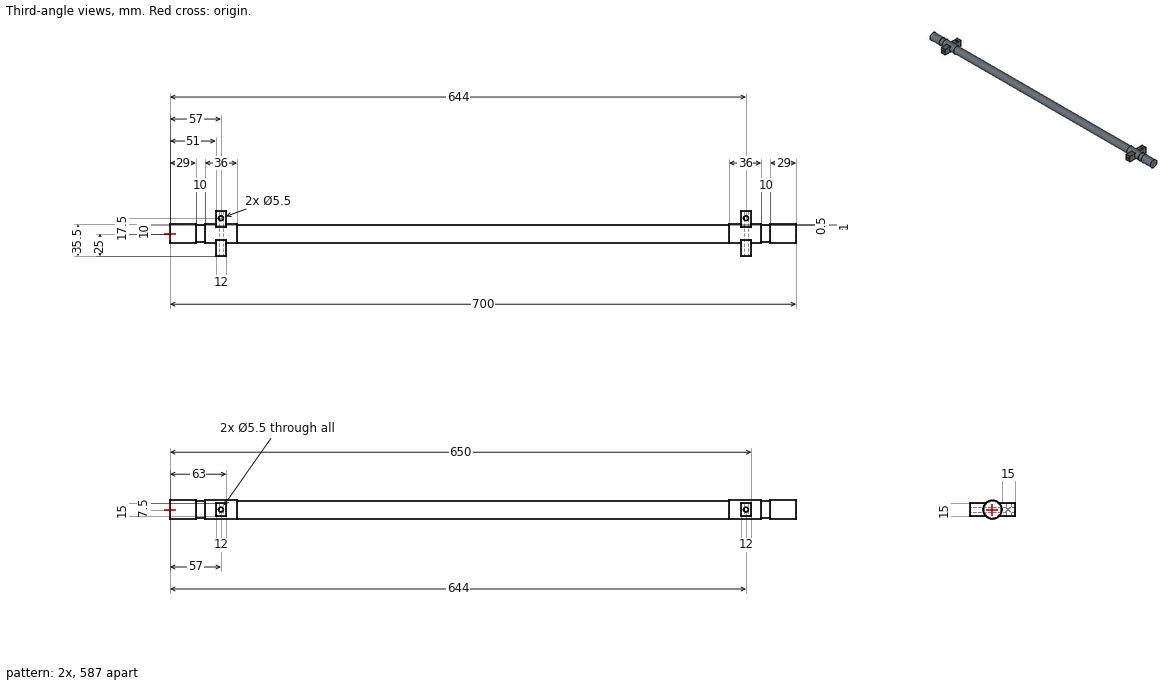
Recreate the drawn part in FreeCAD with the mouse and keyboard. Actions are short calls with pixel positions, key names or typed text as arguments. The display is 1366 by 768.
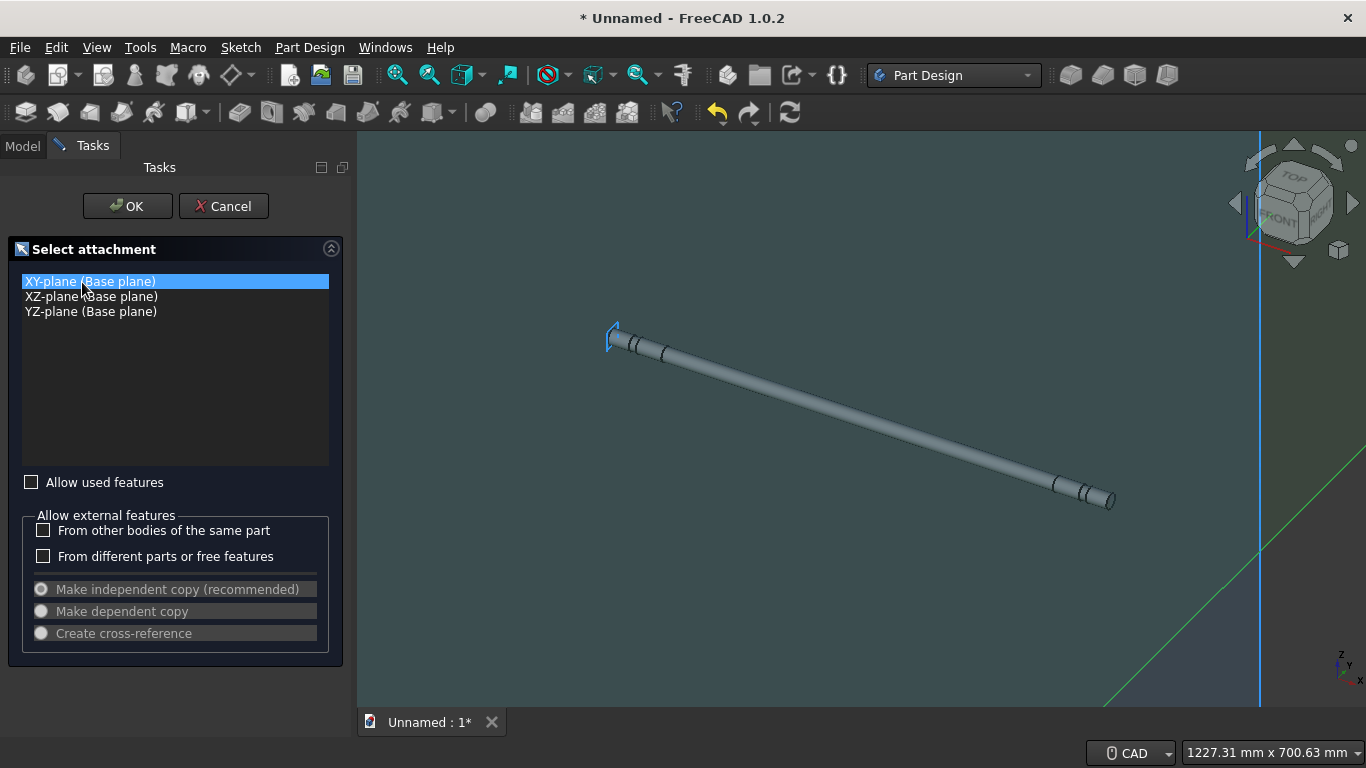
click(128, 206)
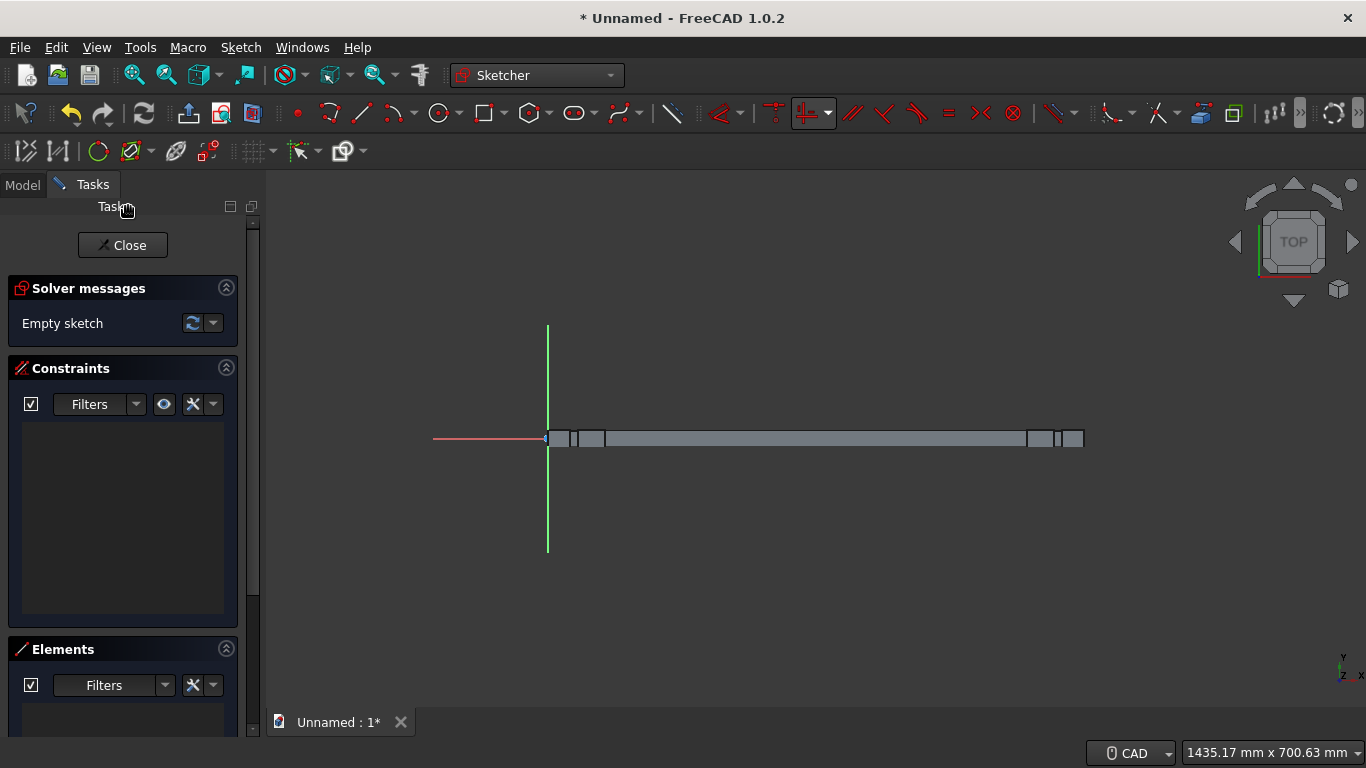
click(254, 114)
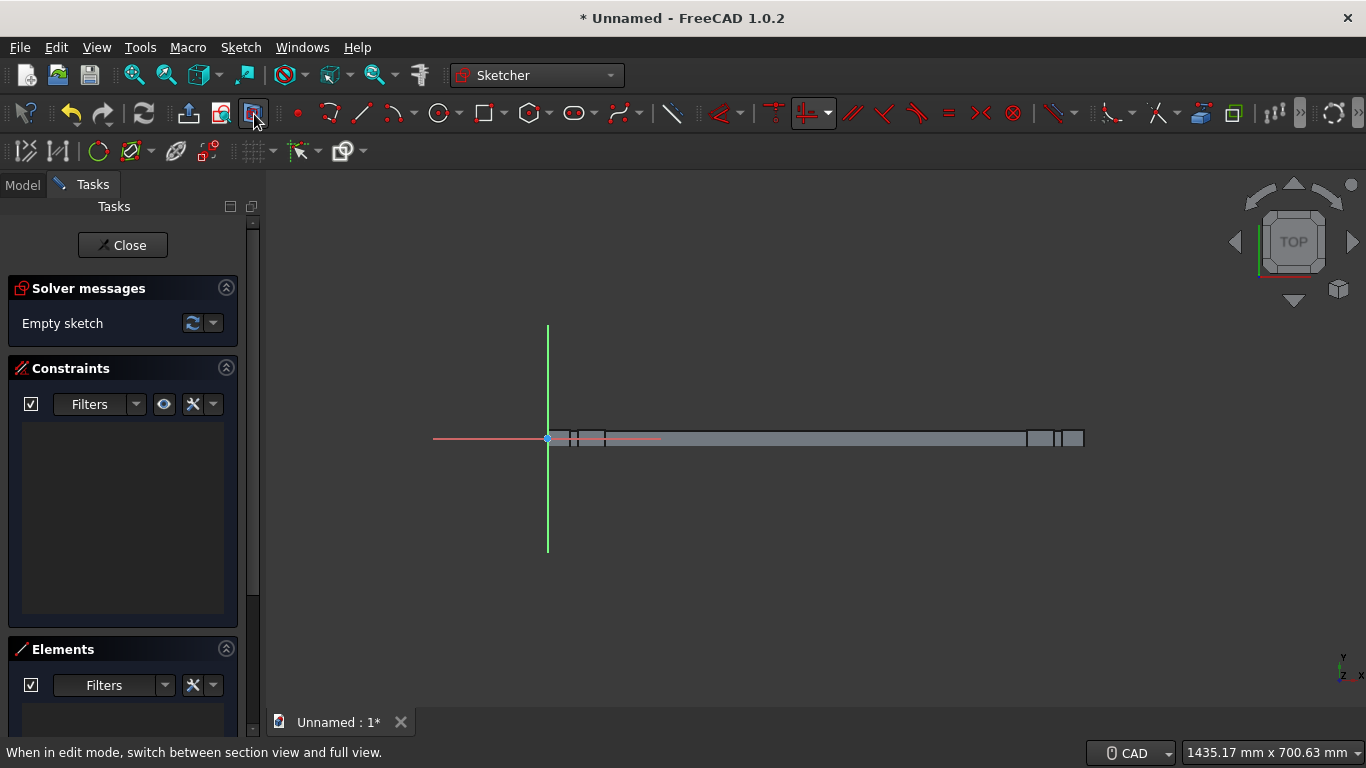
scroll(558, 445, up, 13)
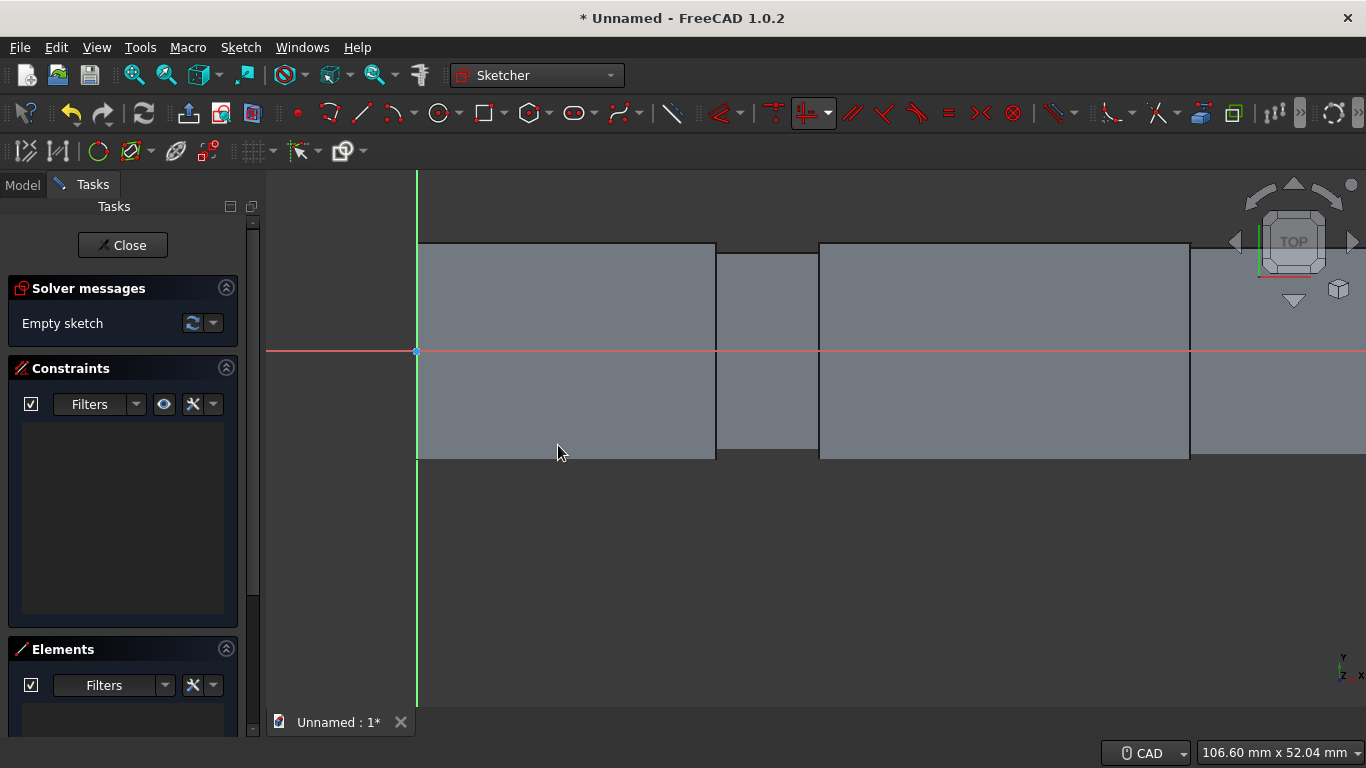
click(484, 114)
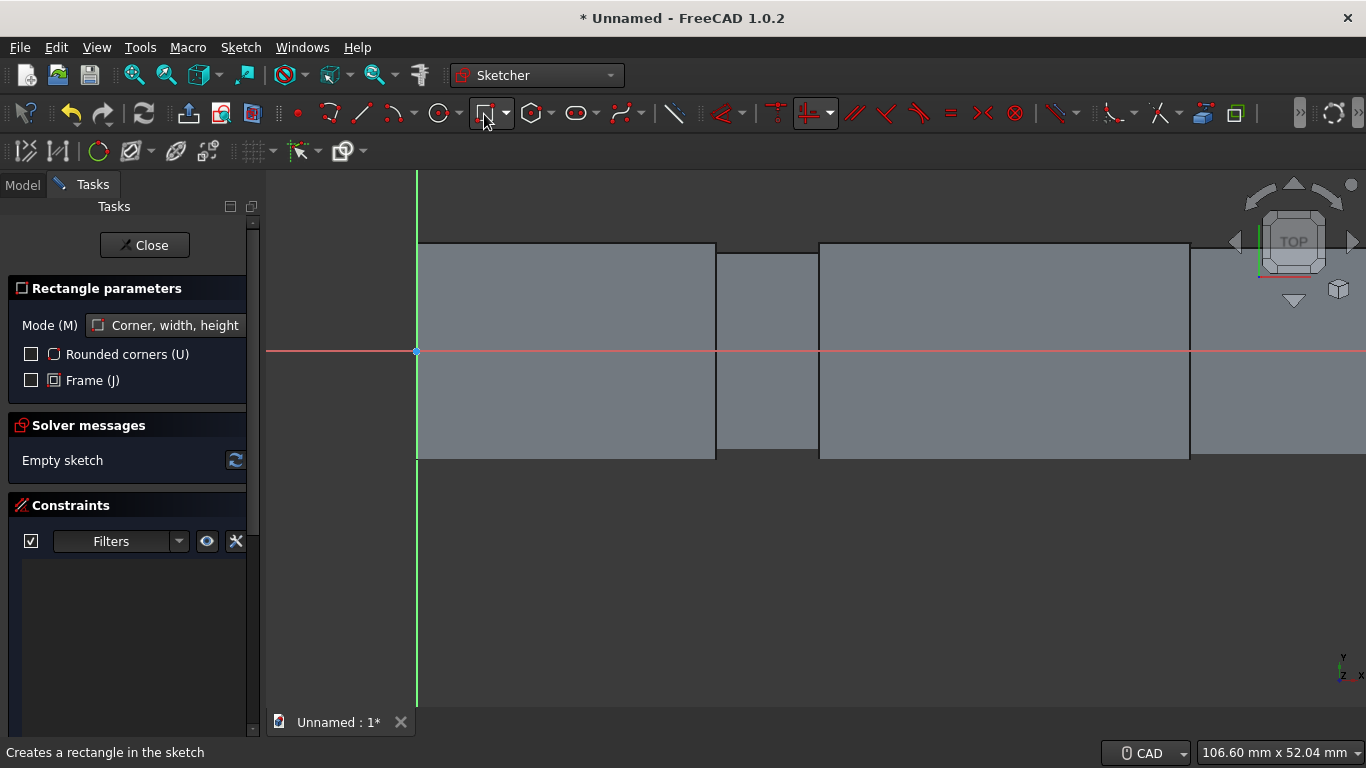
click(943, 243)
click(1067, 609)
key(Escape)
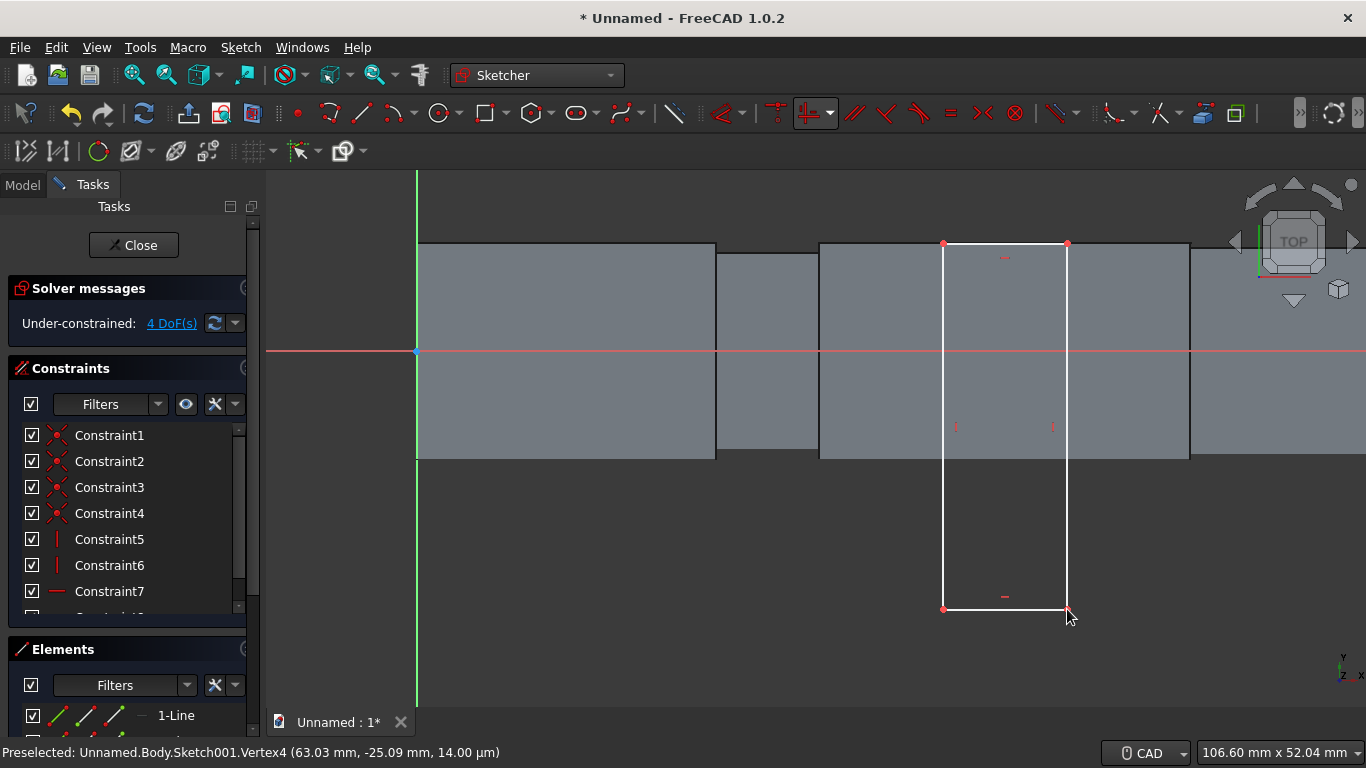
click(722, 114)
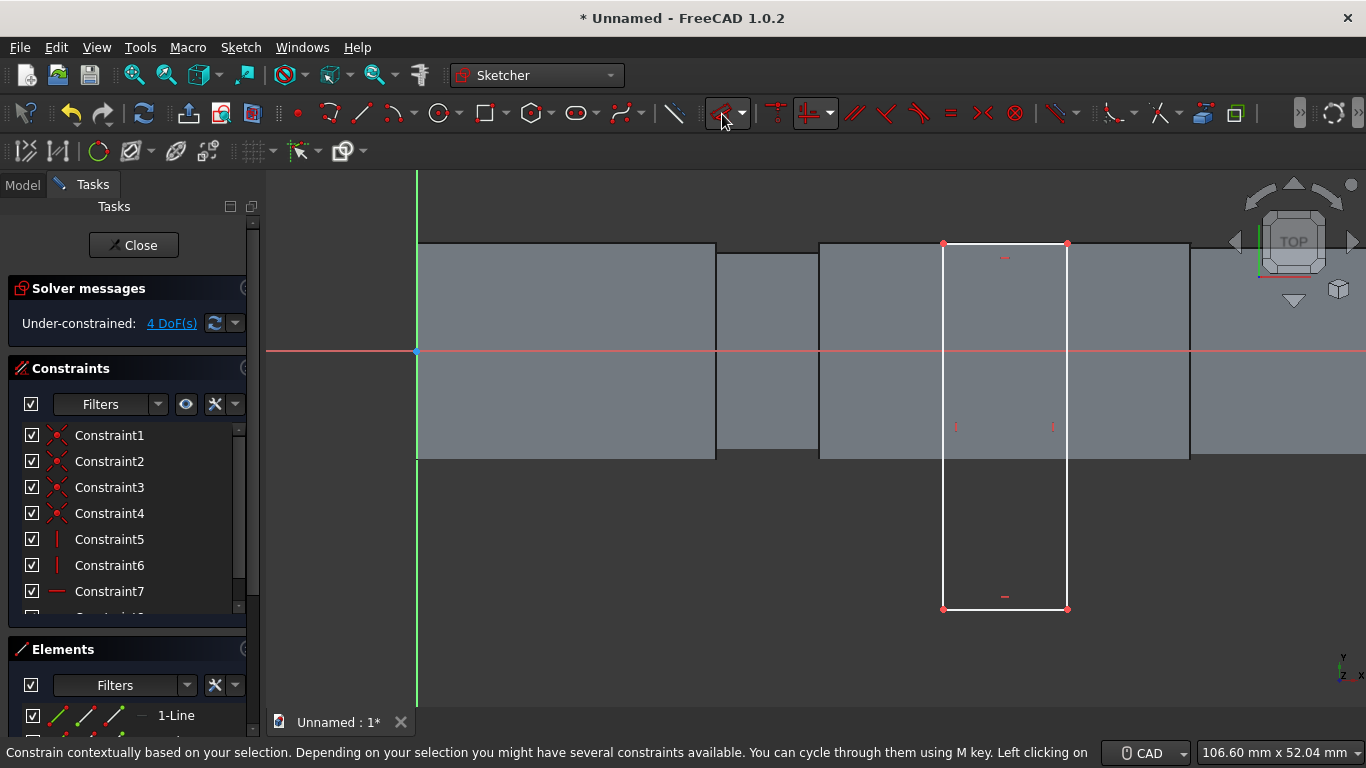
click(980, 610)
click(1005, 644)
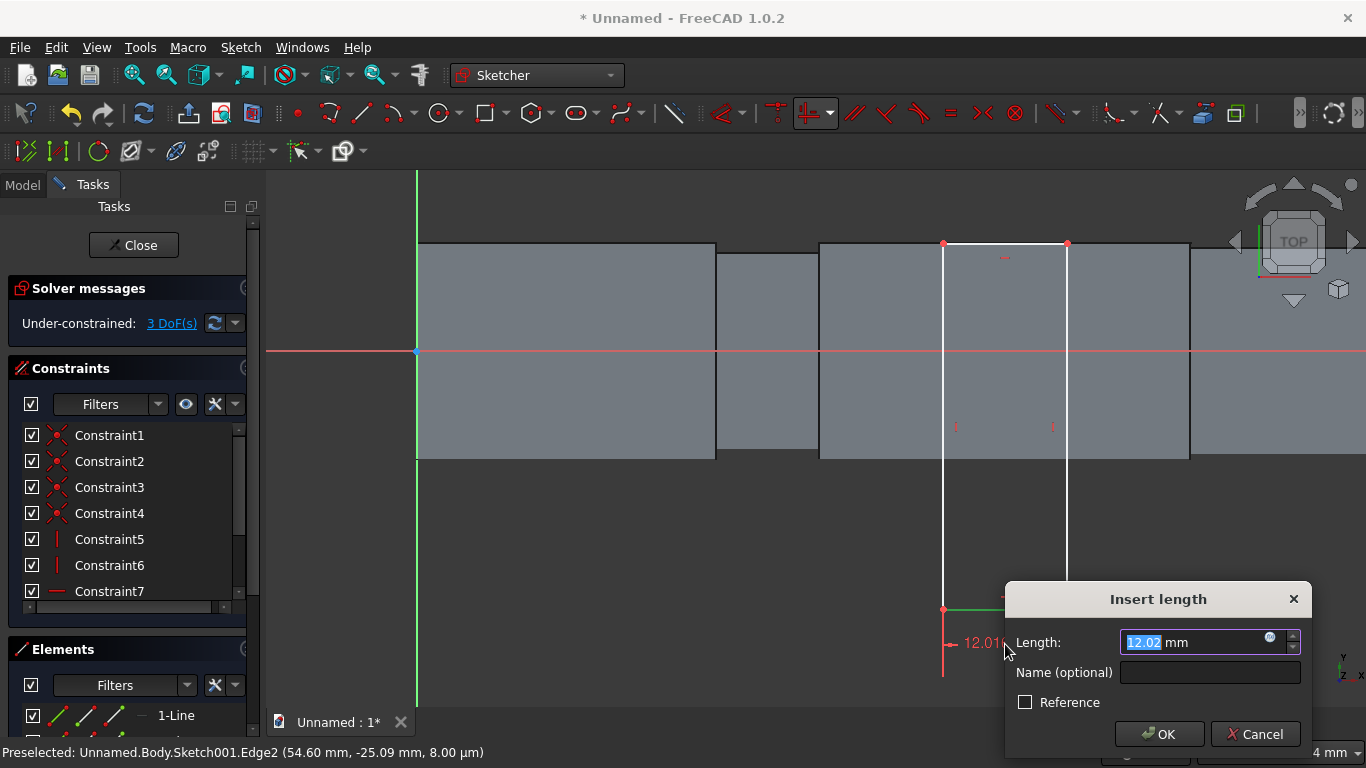
text(12)
key(Return)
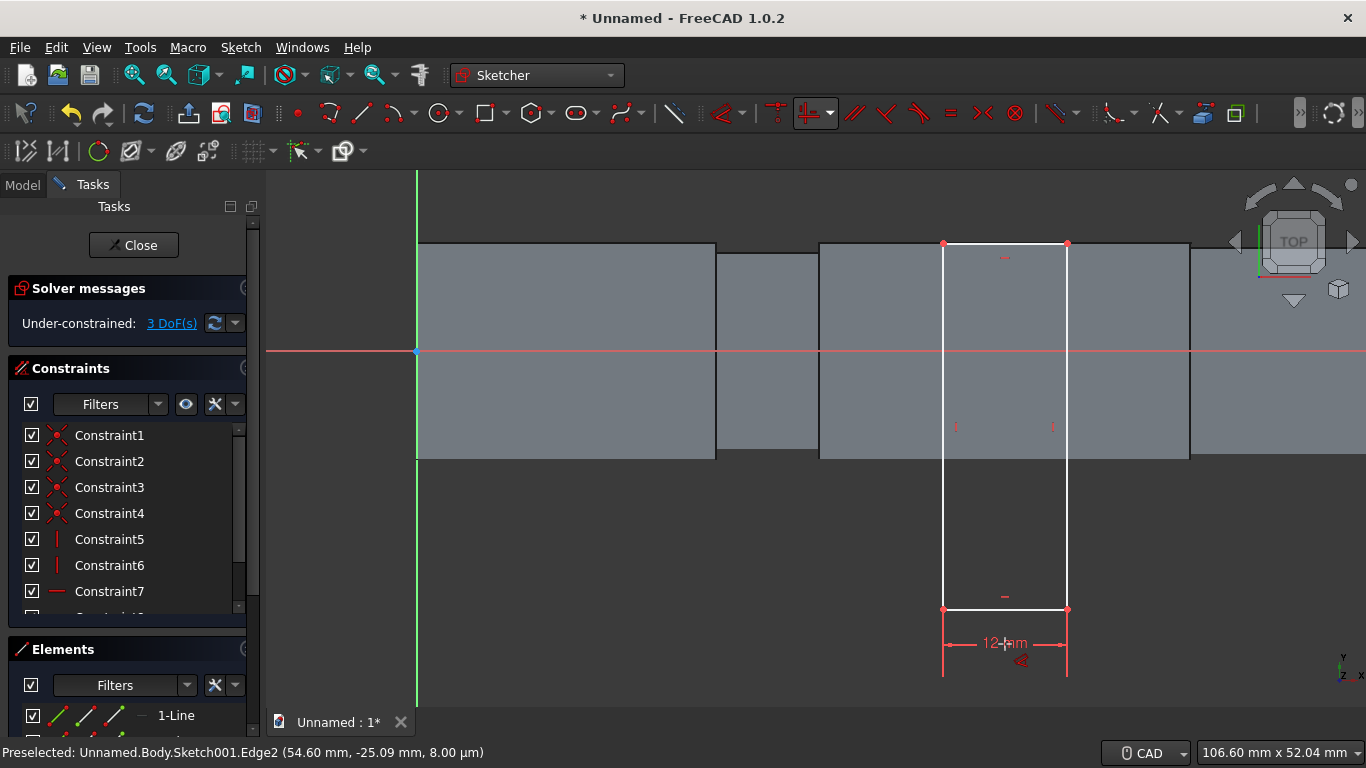
click(943, 244)
click(680, 210)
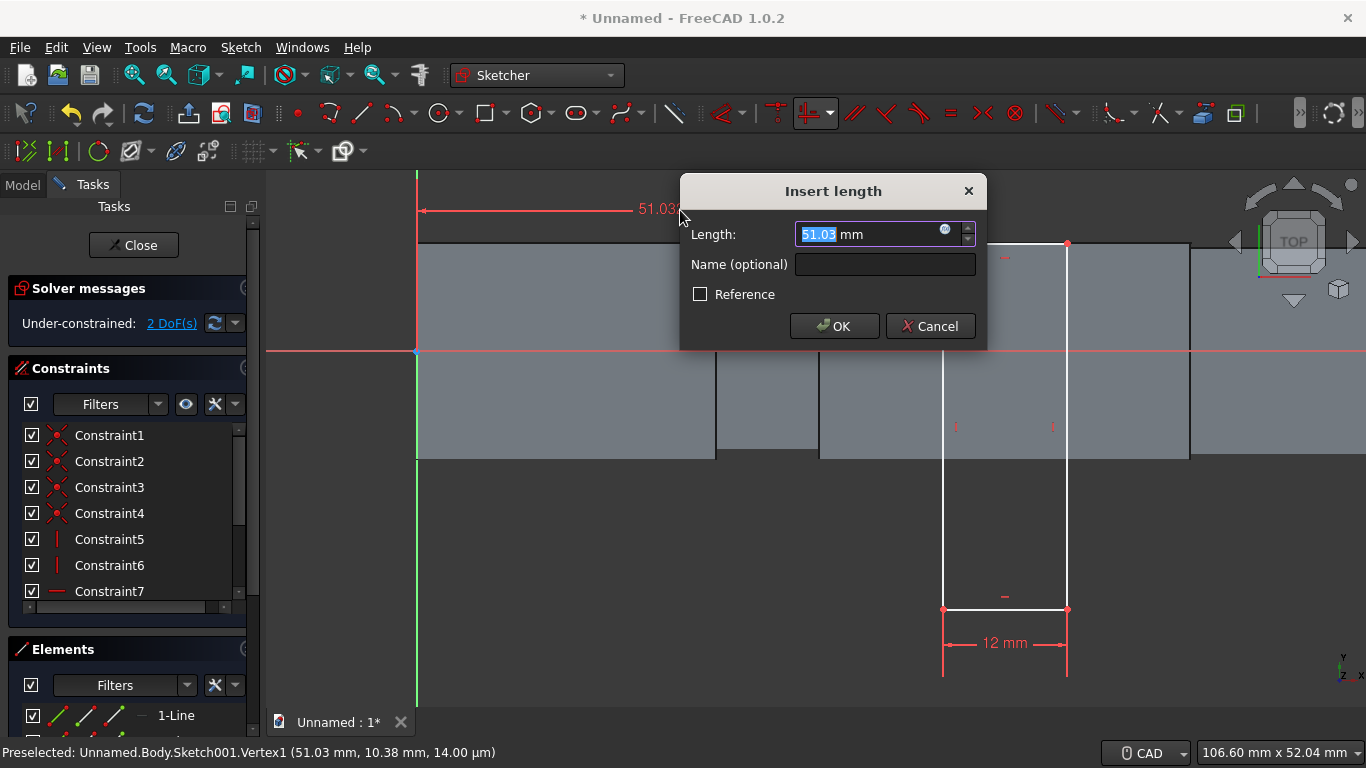
text(51)
key(Return)